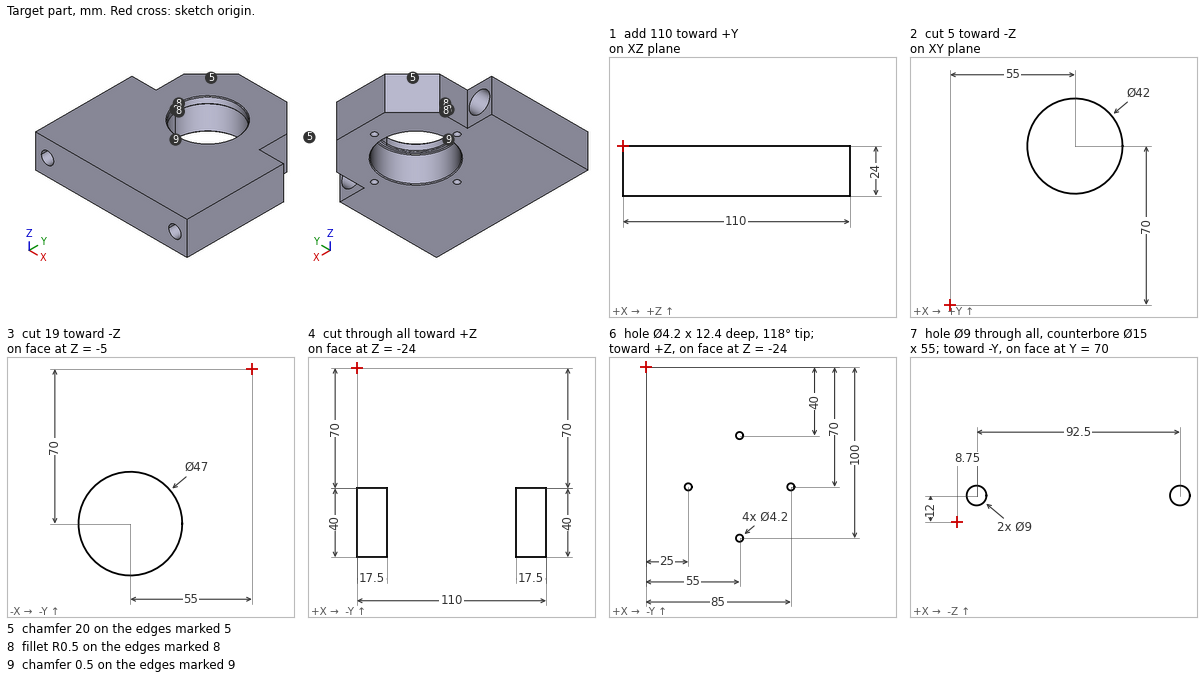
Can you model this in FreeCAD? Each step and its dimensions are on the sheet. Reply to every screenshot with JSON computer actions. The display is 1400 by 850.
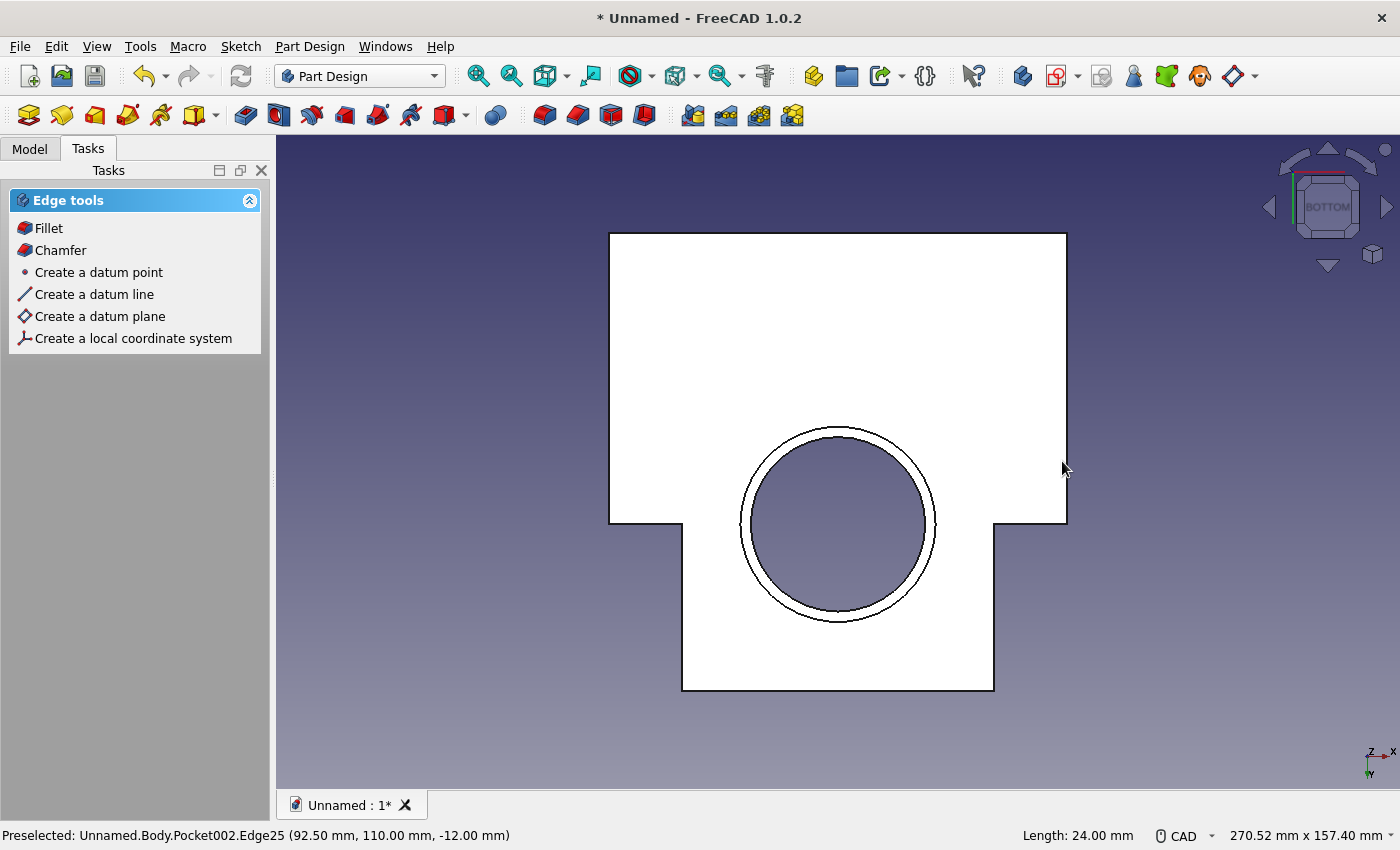
{"action": "key", "text": "4"}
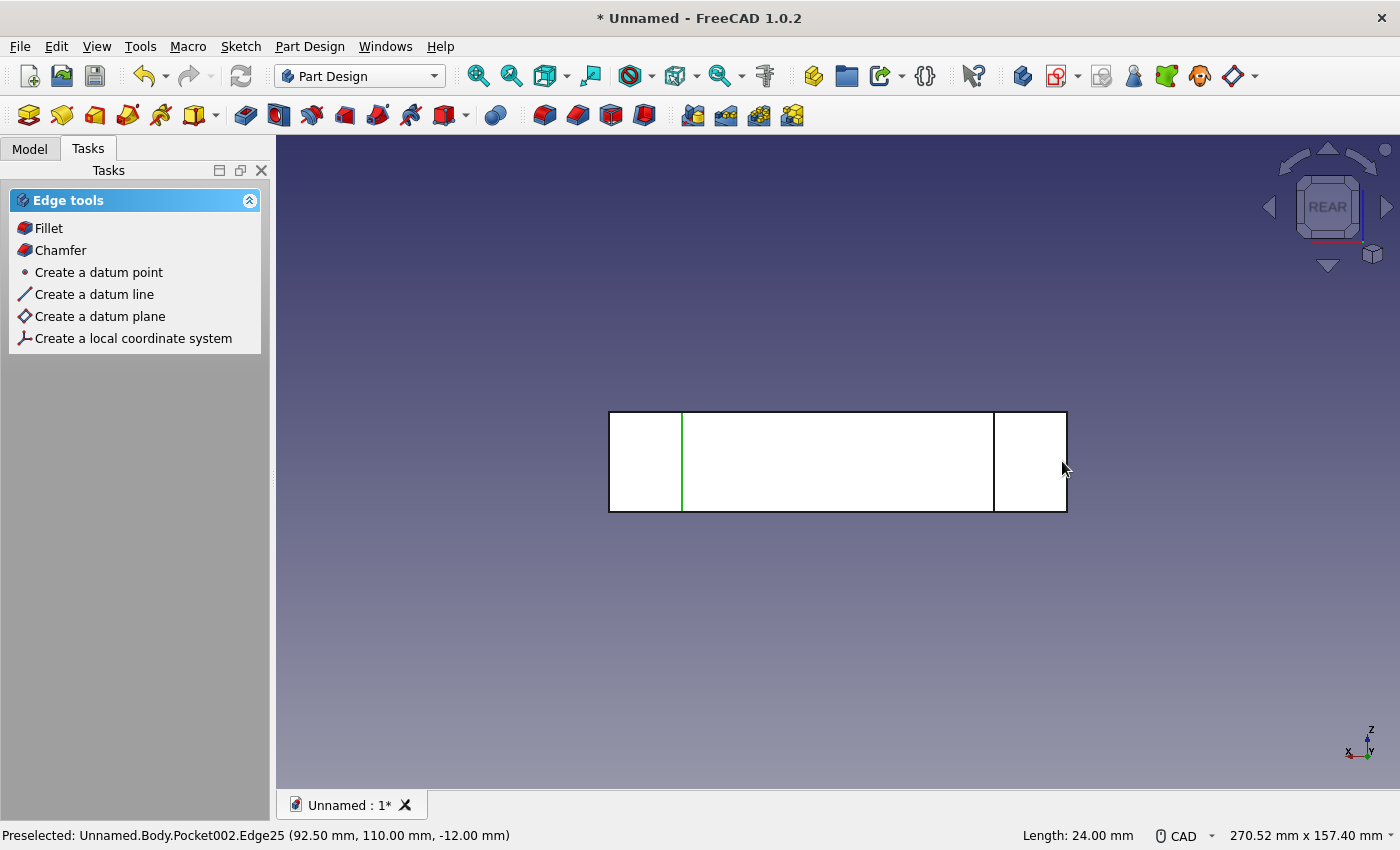
{"action": "left_click", "coordinate": [479, 76]}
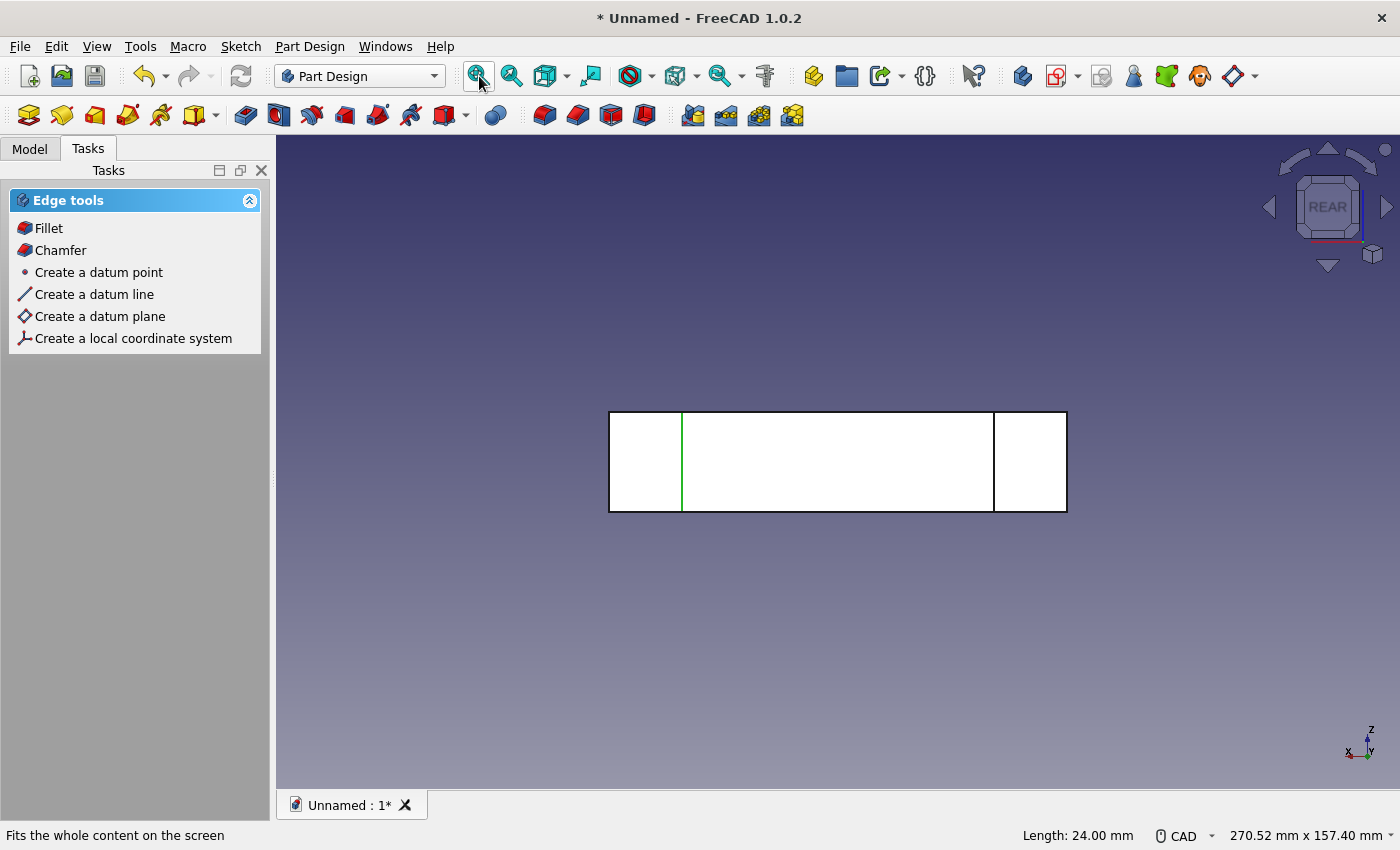
{"action": "left_click", "coordinate": [994, 461], "text": "ctrl"}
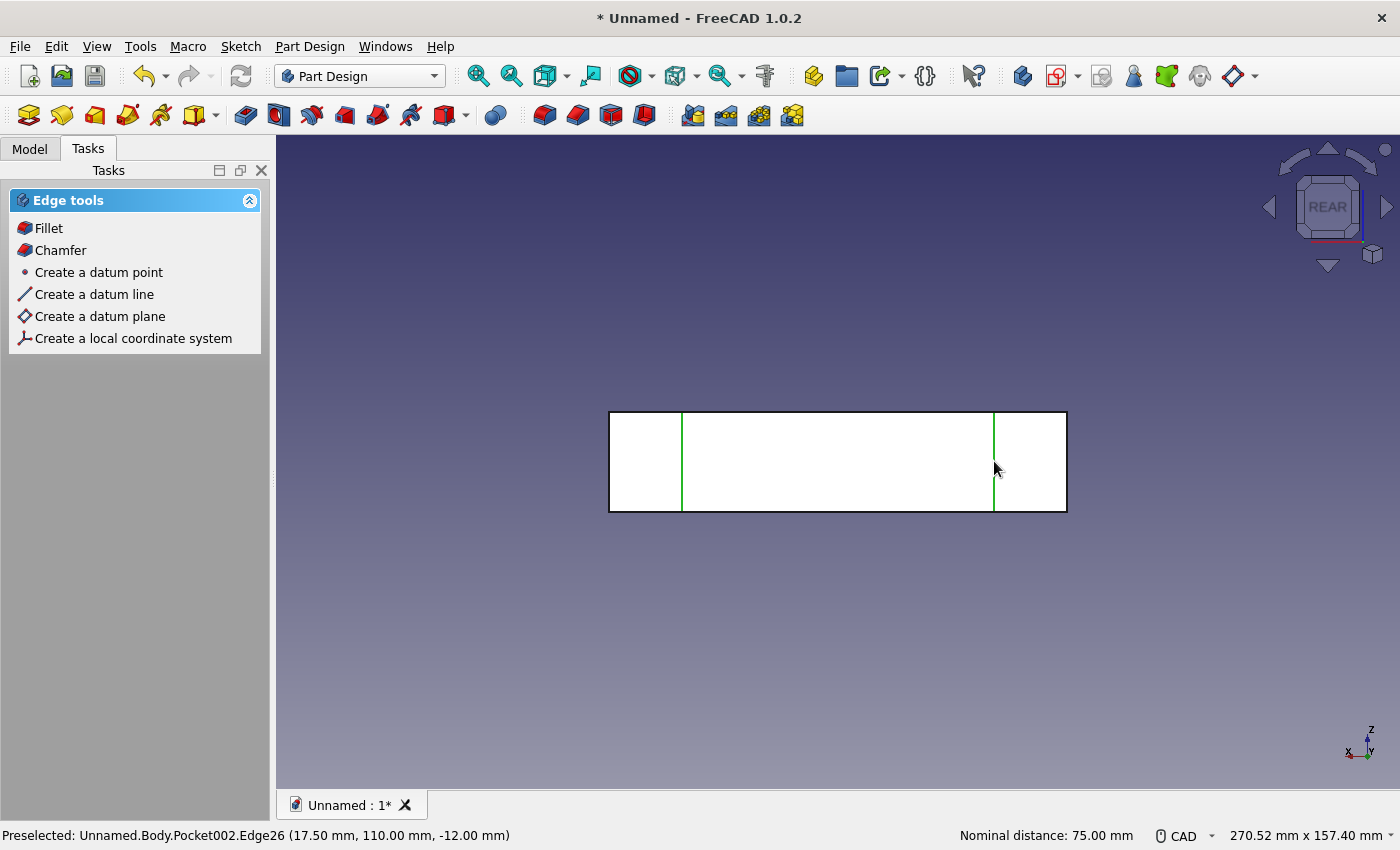
{"action": "left_click", "coordinate": [578, 116]}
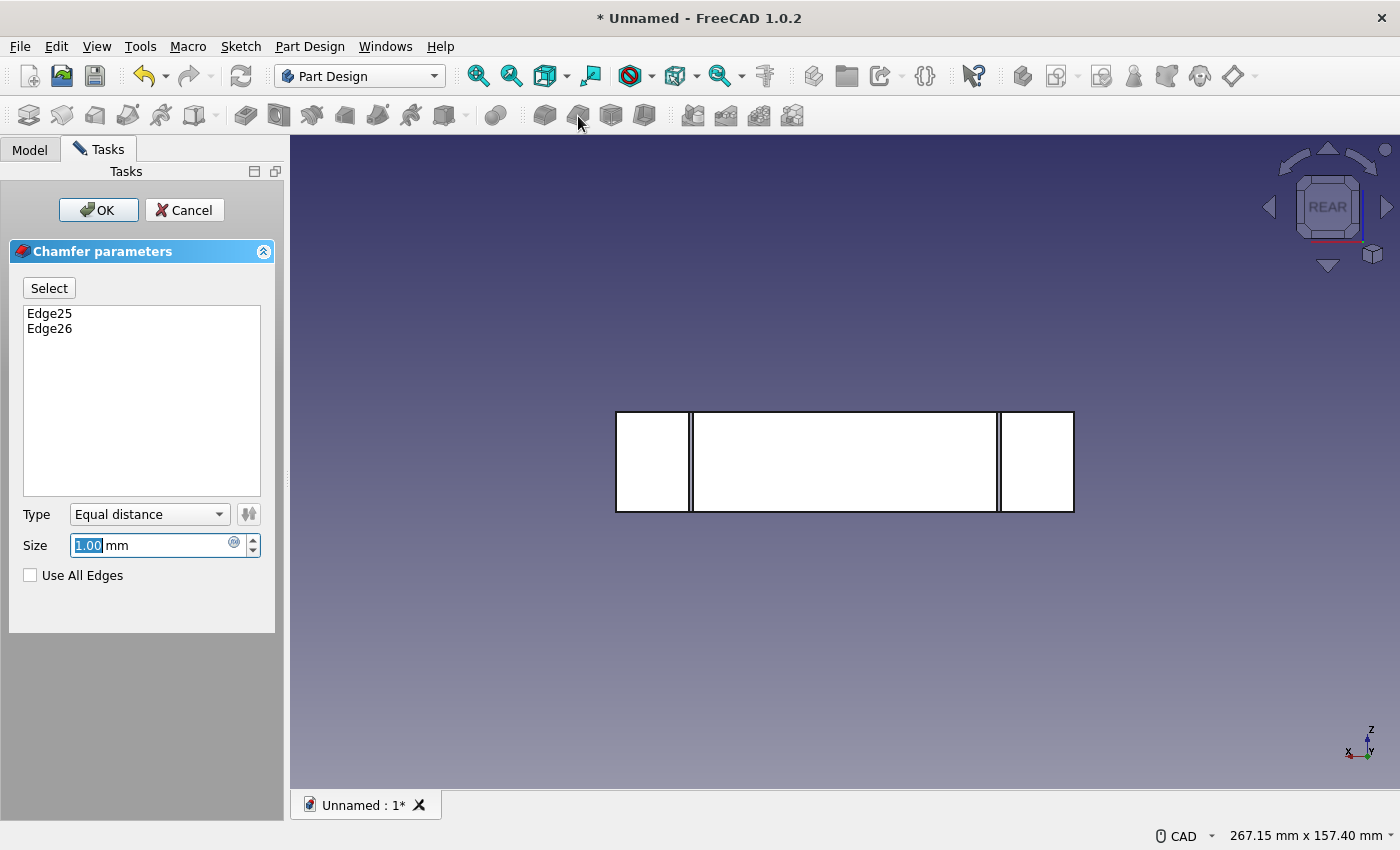
{"action": "type", "text": "20"}
{"action": "key", "text": "Tab"}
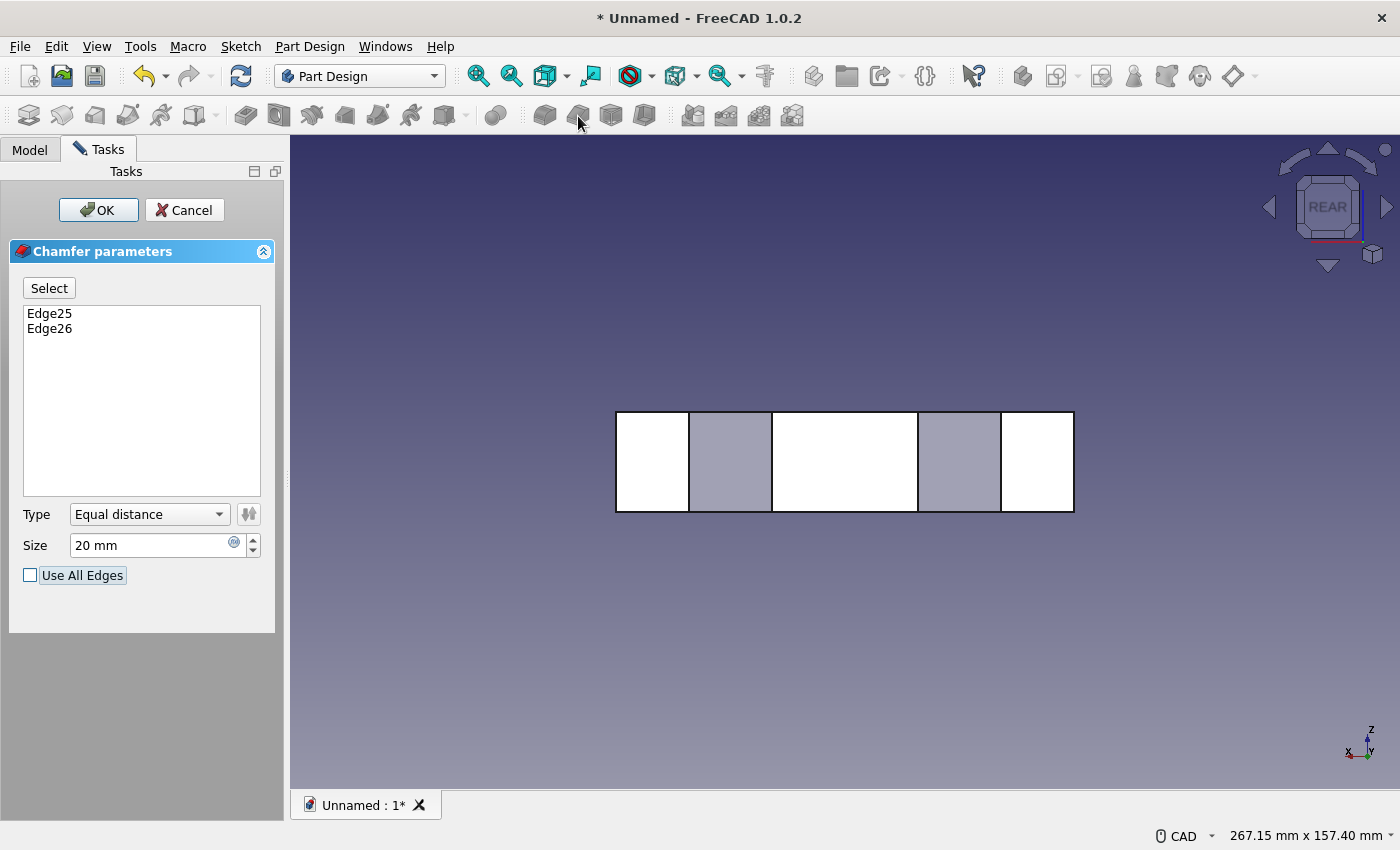
{"action": "left_click", "coordinate": [99, 210]}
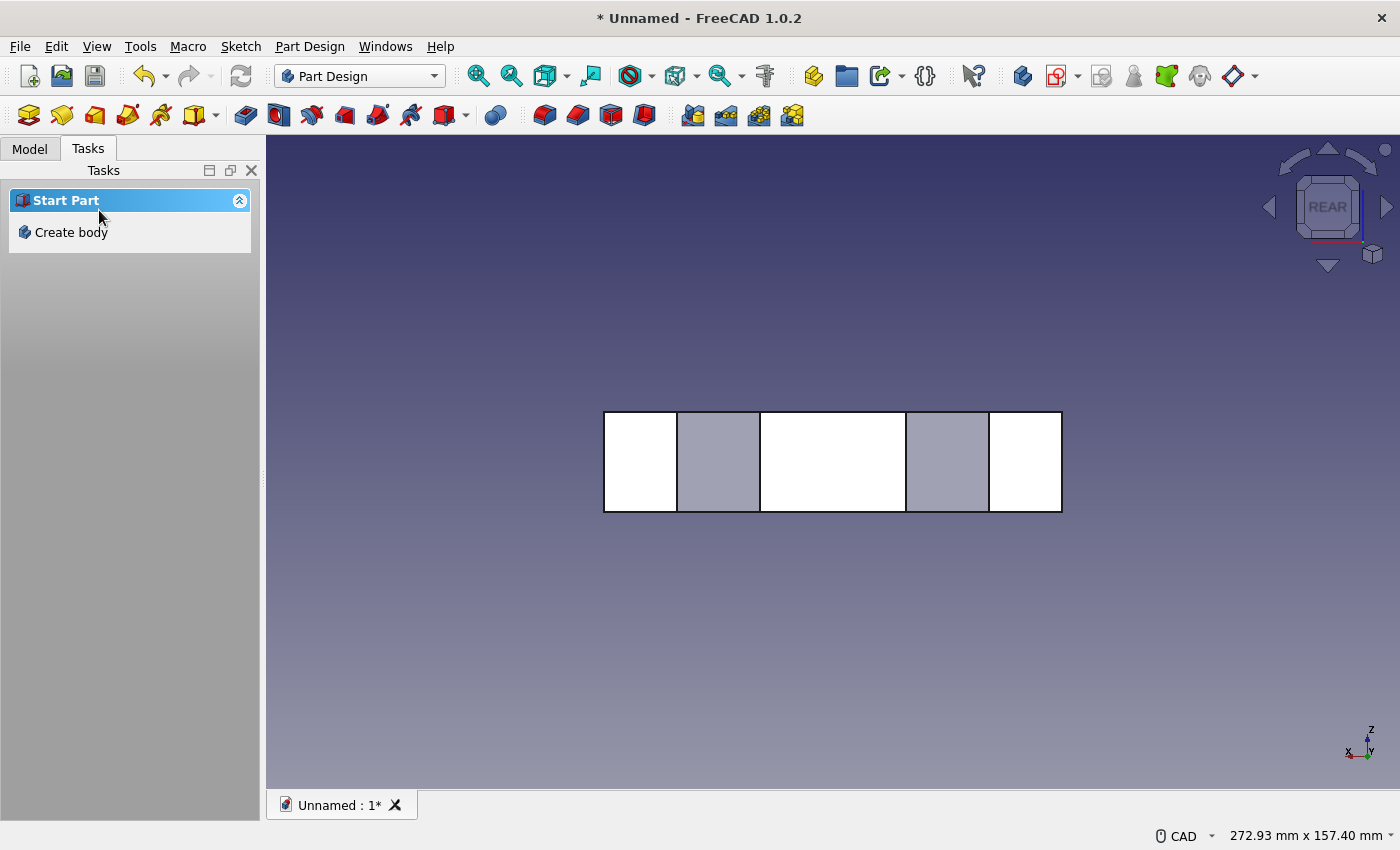
{"action": "left_click", "coordinate": [479, 76]}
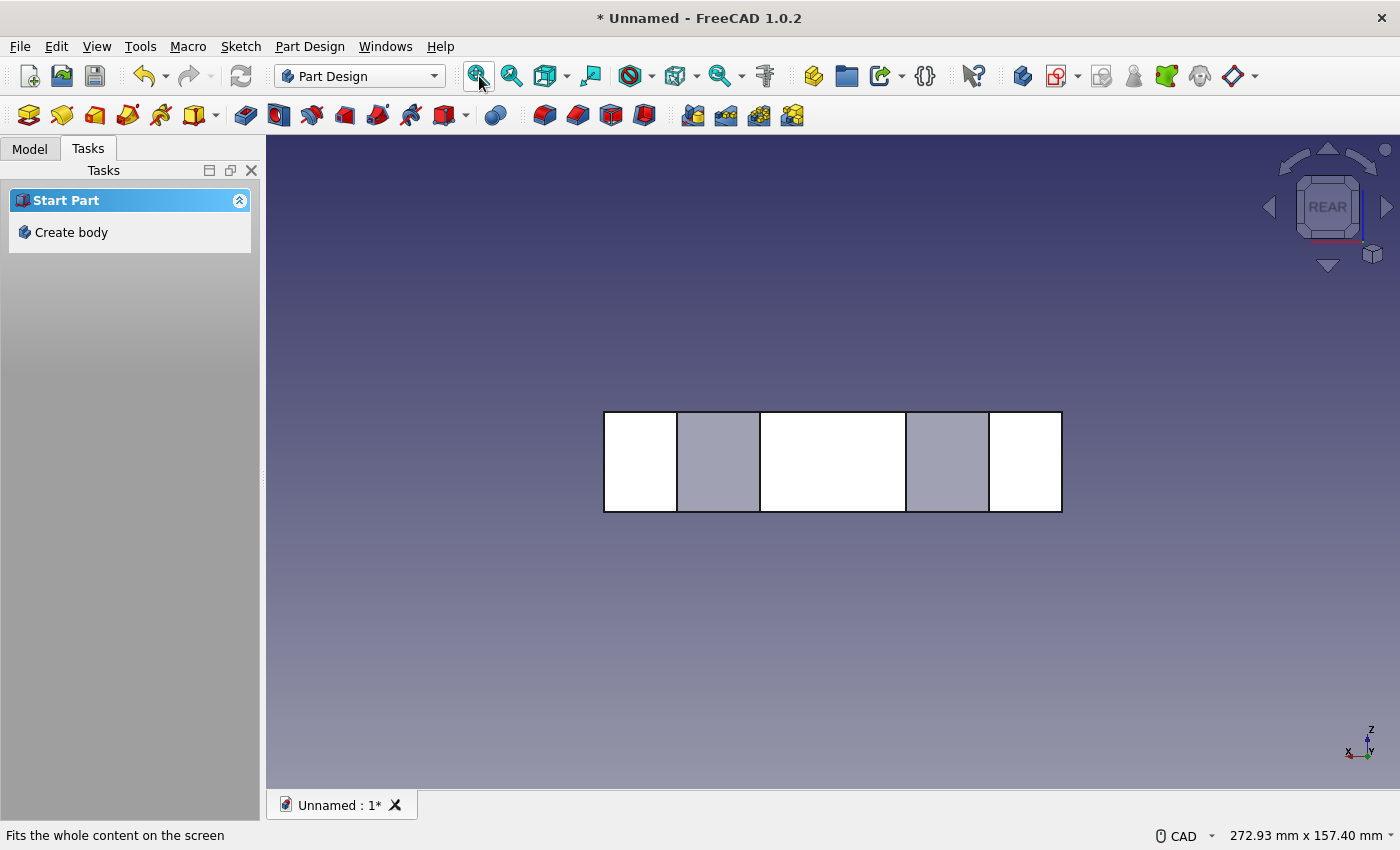
{"action": "key", "text": "5"}